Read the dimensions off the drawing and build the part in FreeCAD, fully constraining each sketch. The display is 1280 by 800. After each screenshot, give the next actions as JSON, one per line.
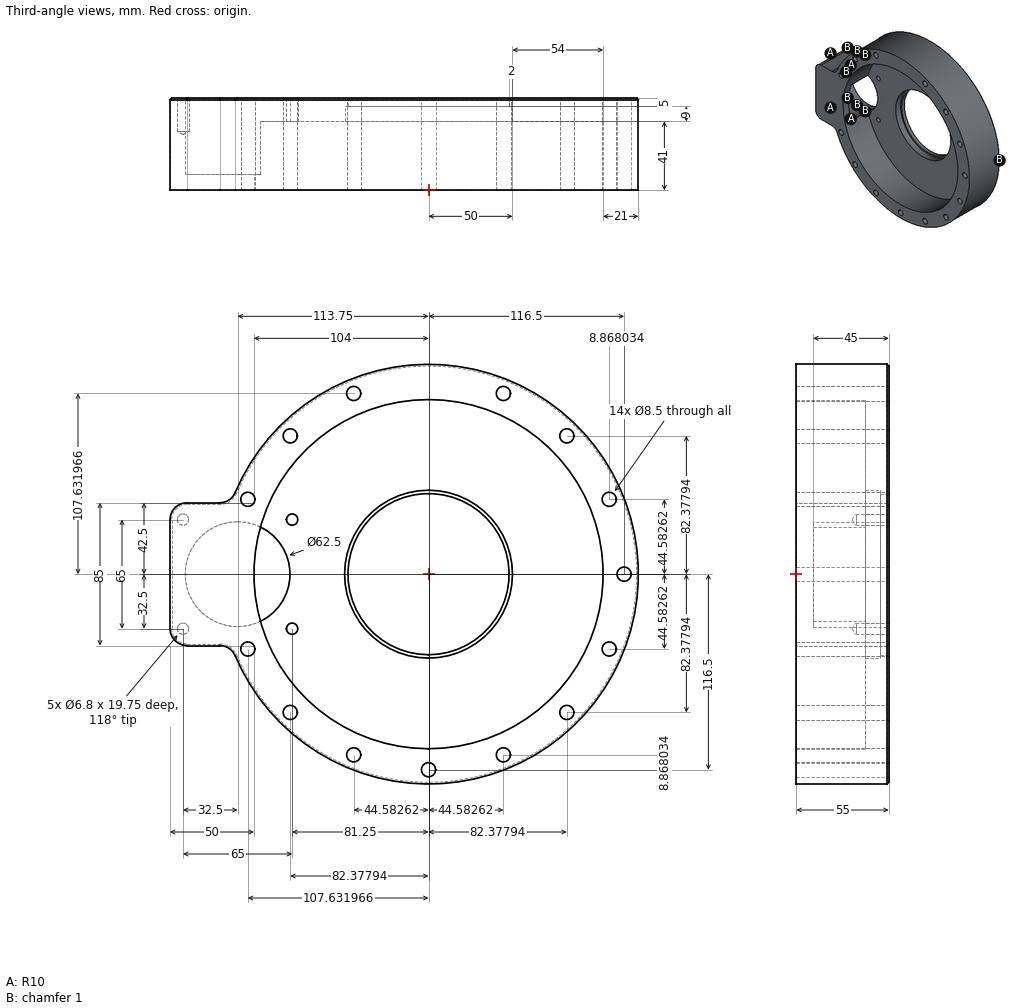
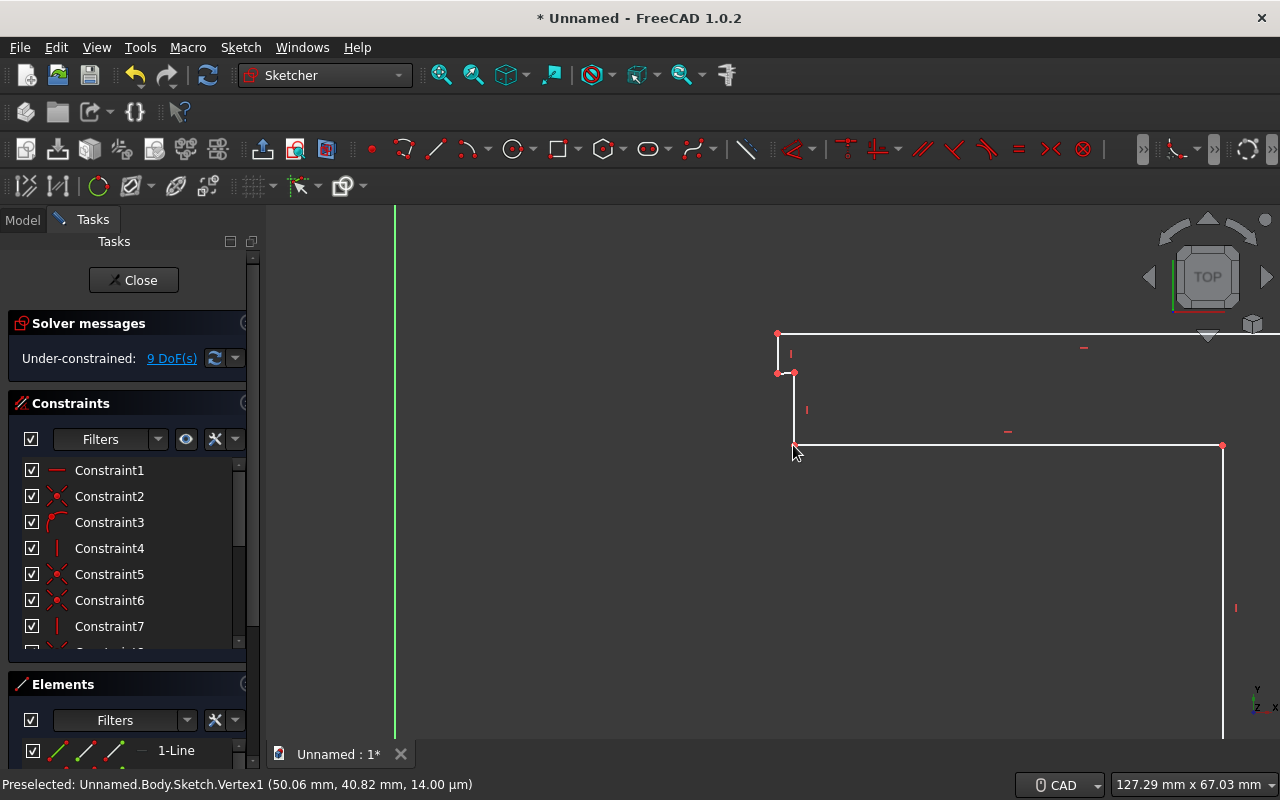
{"action": "scroll", "coordinate": [475, 376], "scroll_direction": "down", "scroll_amount": 3}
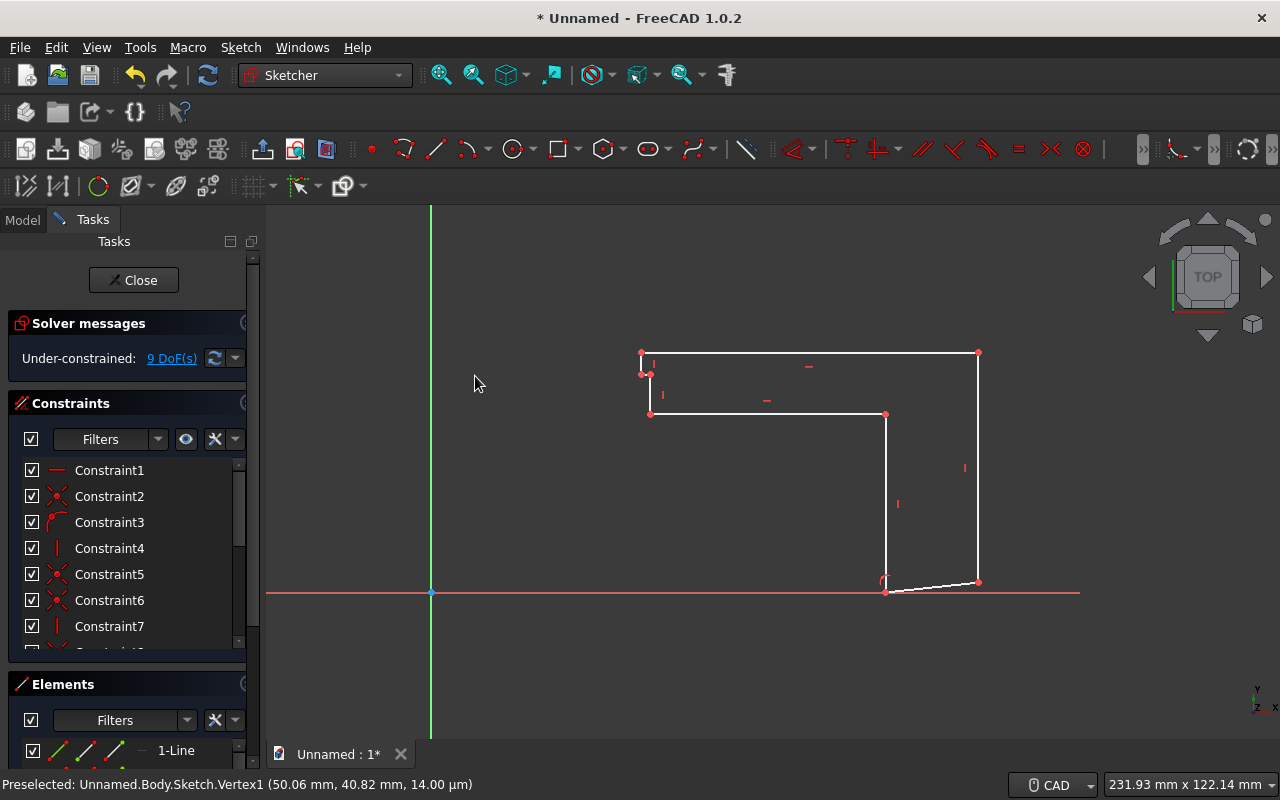
{"action": "scroll", "coordinate": [951, 586], "scroll_direction": "up", "scroll_amount": 4}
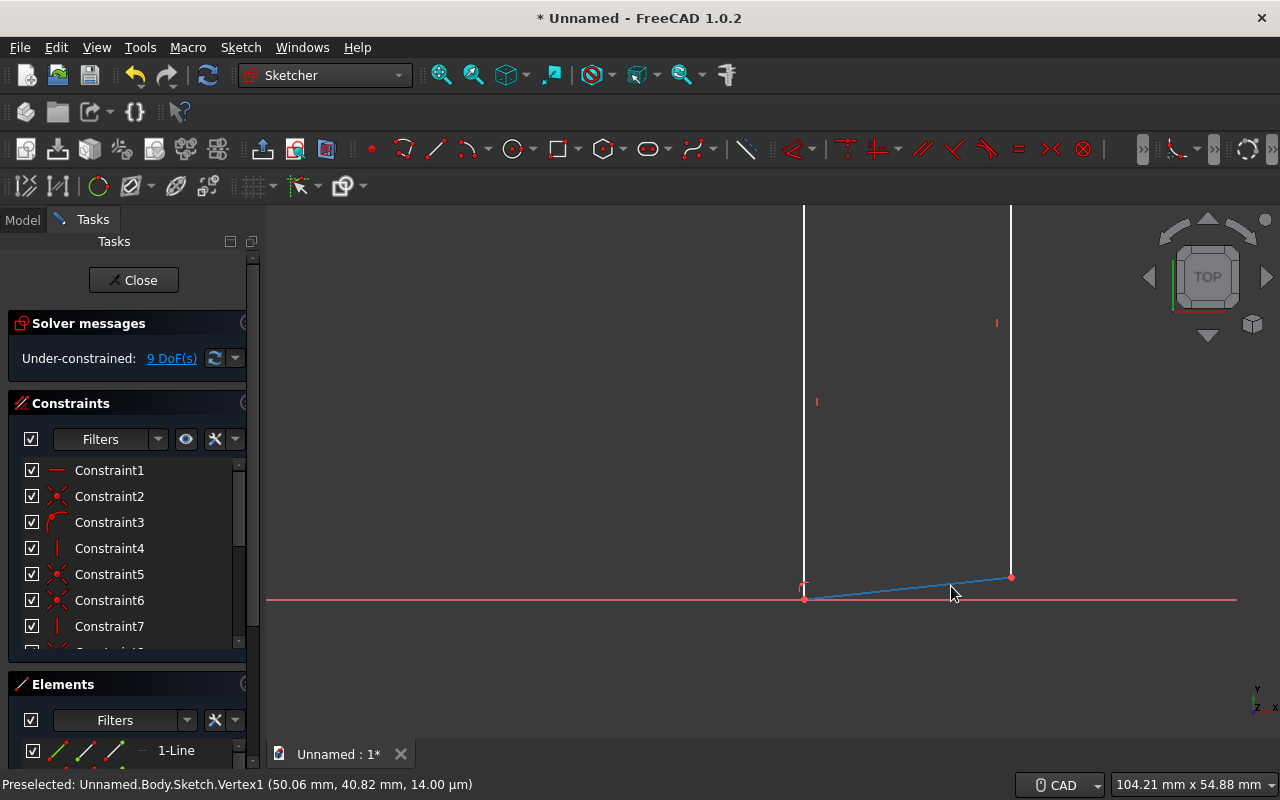
{"action": "left_click", "coordinate": [949, 584]}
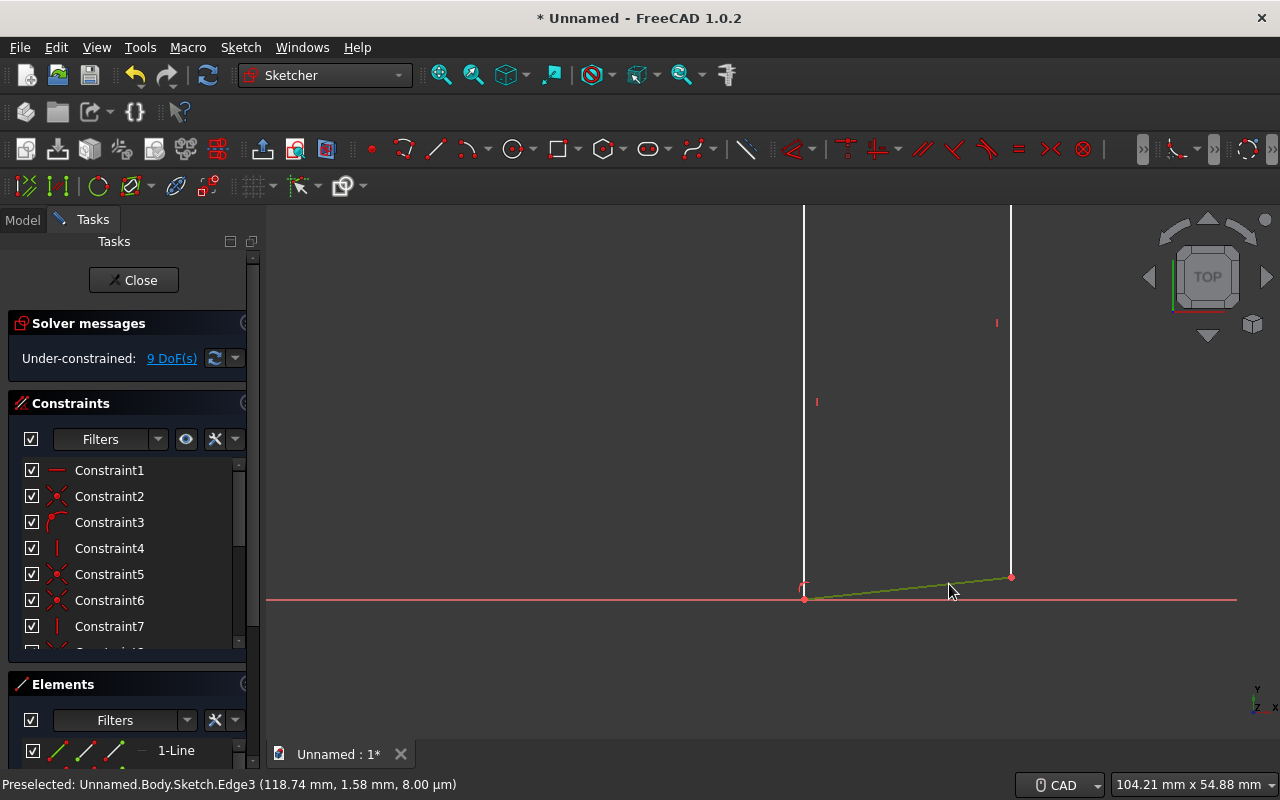
{"action": "key", "text": "h"}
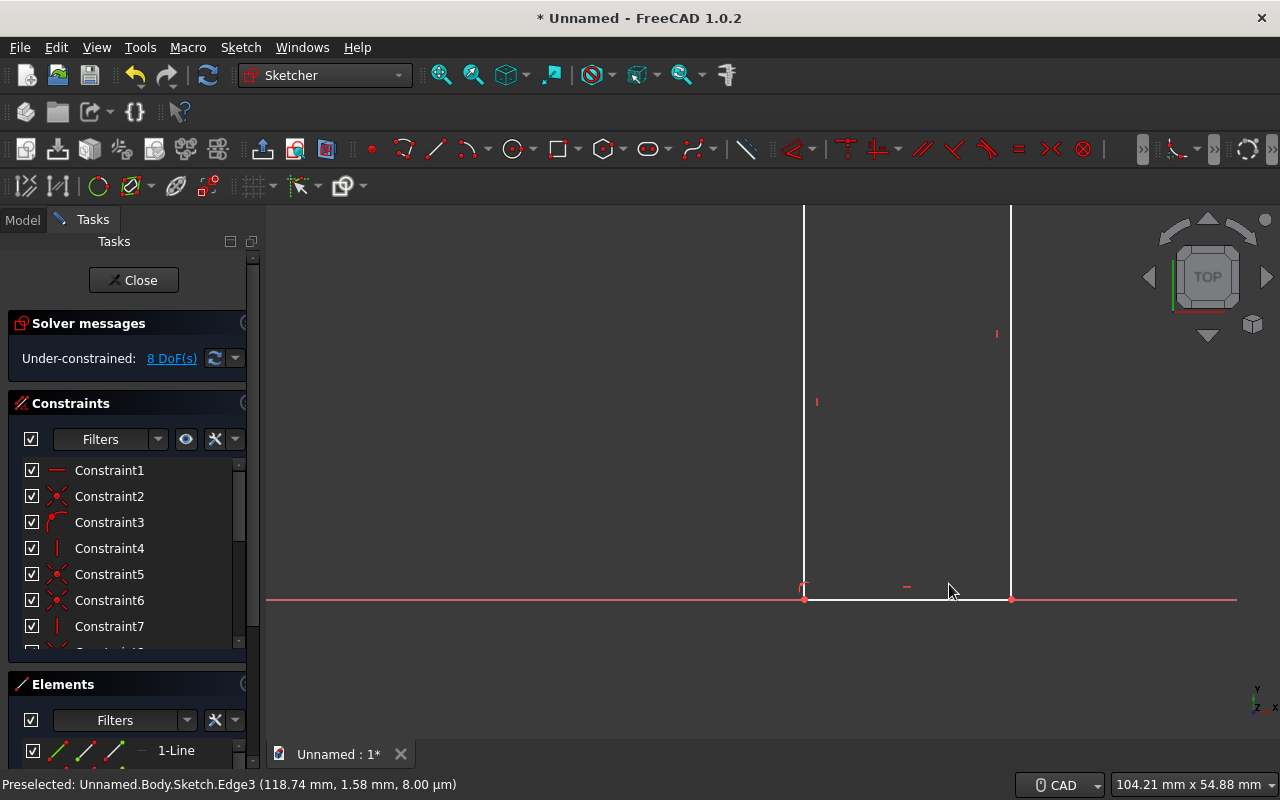
{"action": "scroll", "coordinate": [952, 586], "scroll_direction": "down", "scroll_amount": 4}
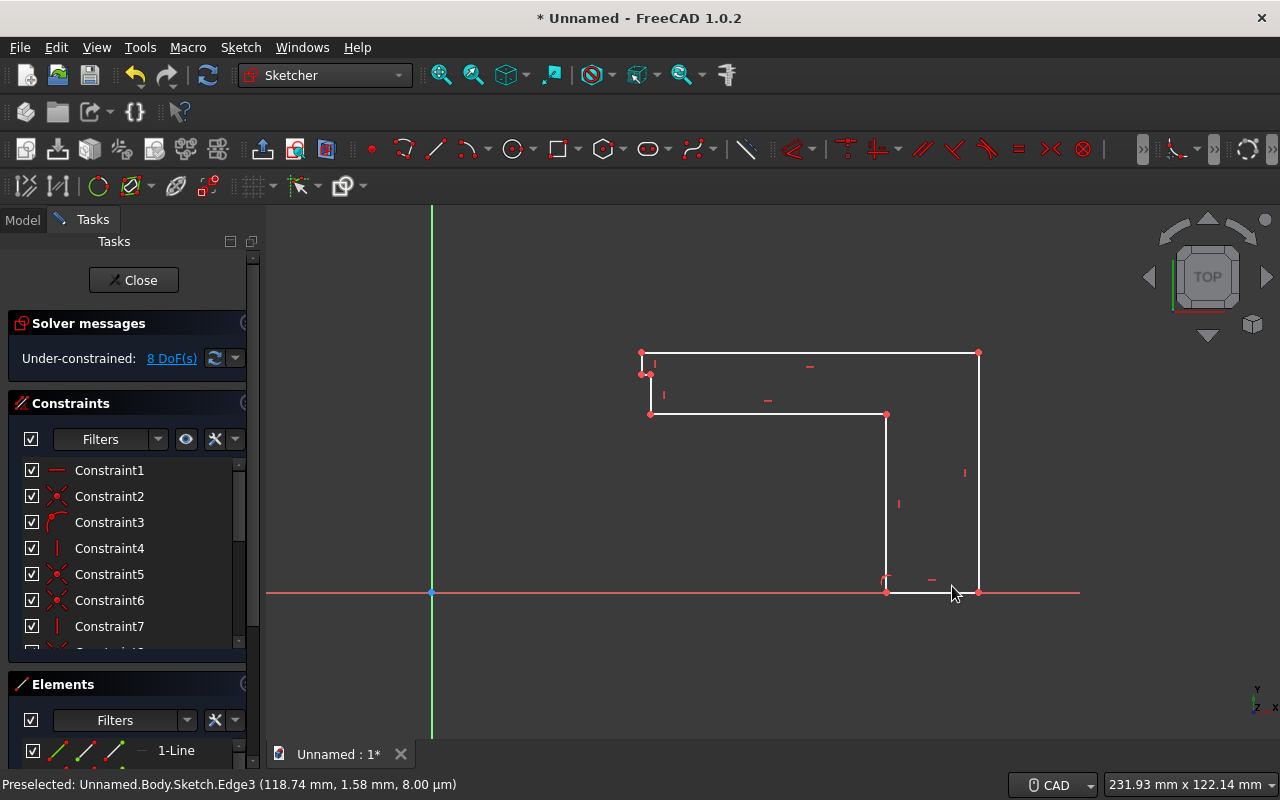
{"action": "scroll", "coordinate": [646, 375], "scroll_direction": "up", "scroll_amount": 6}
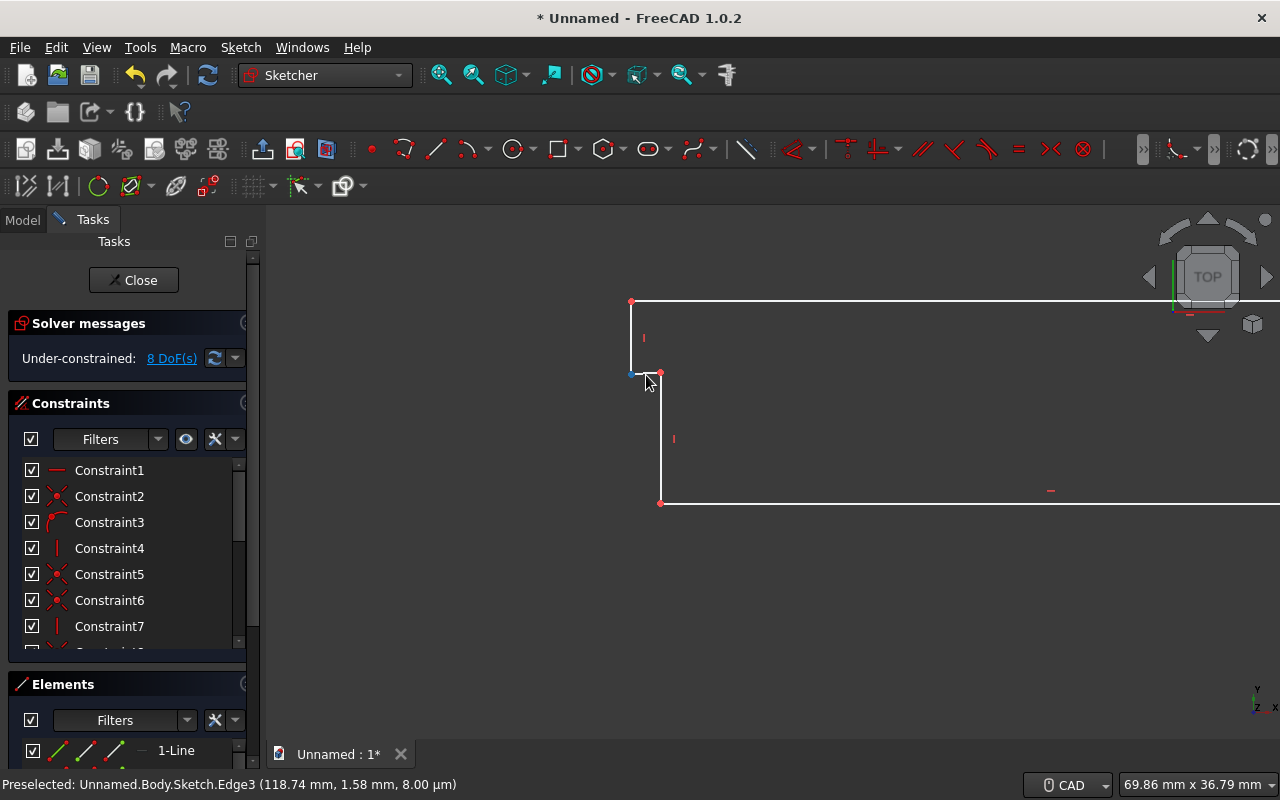
{"action": "left_click", "coordinate": [646, 373]}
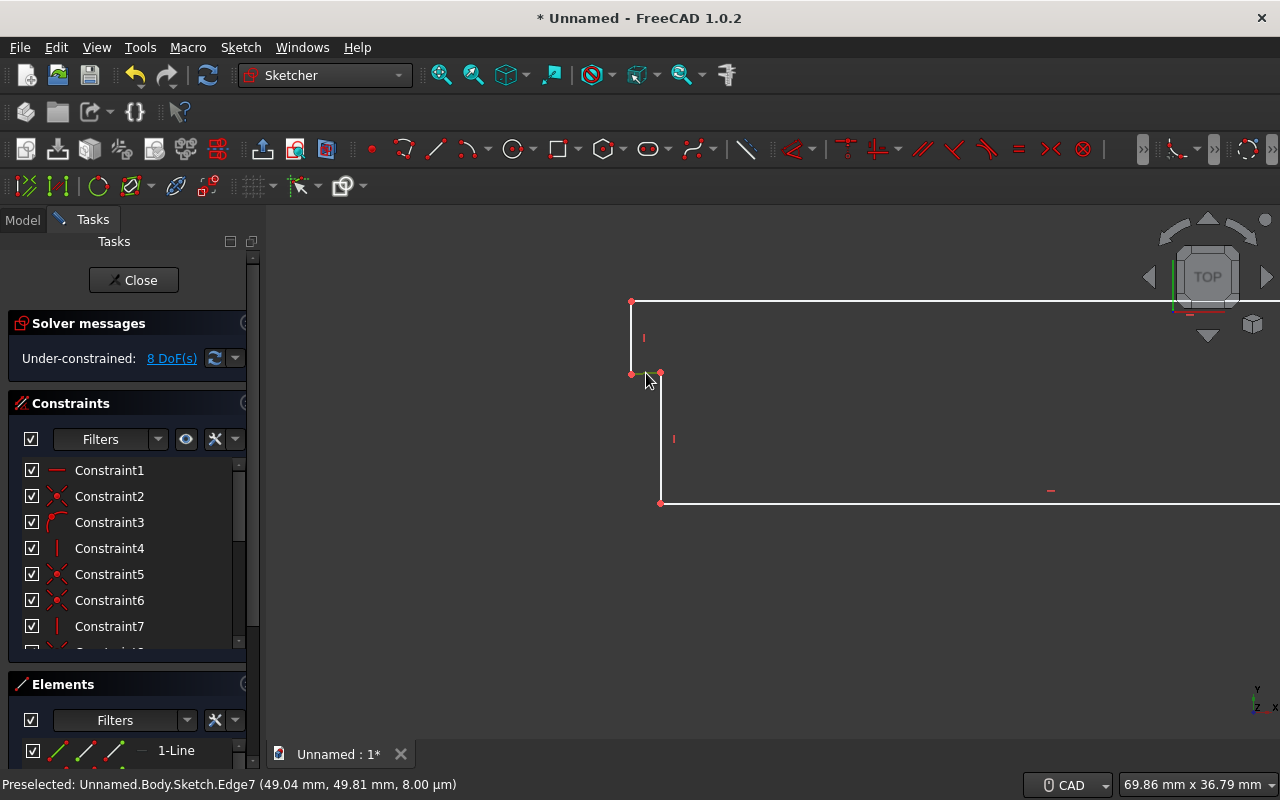
{"action": "left_click", "coordinate": [900, 150]}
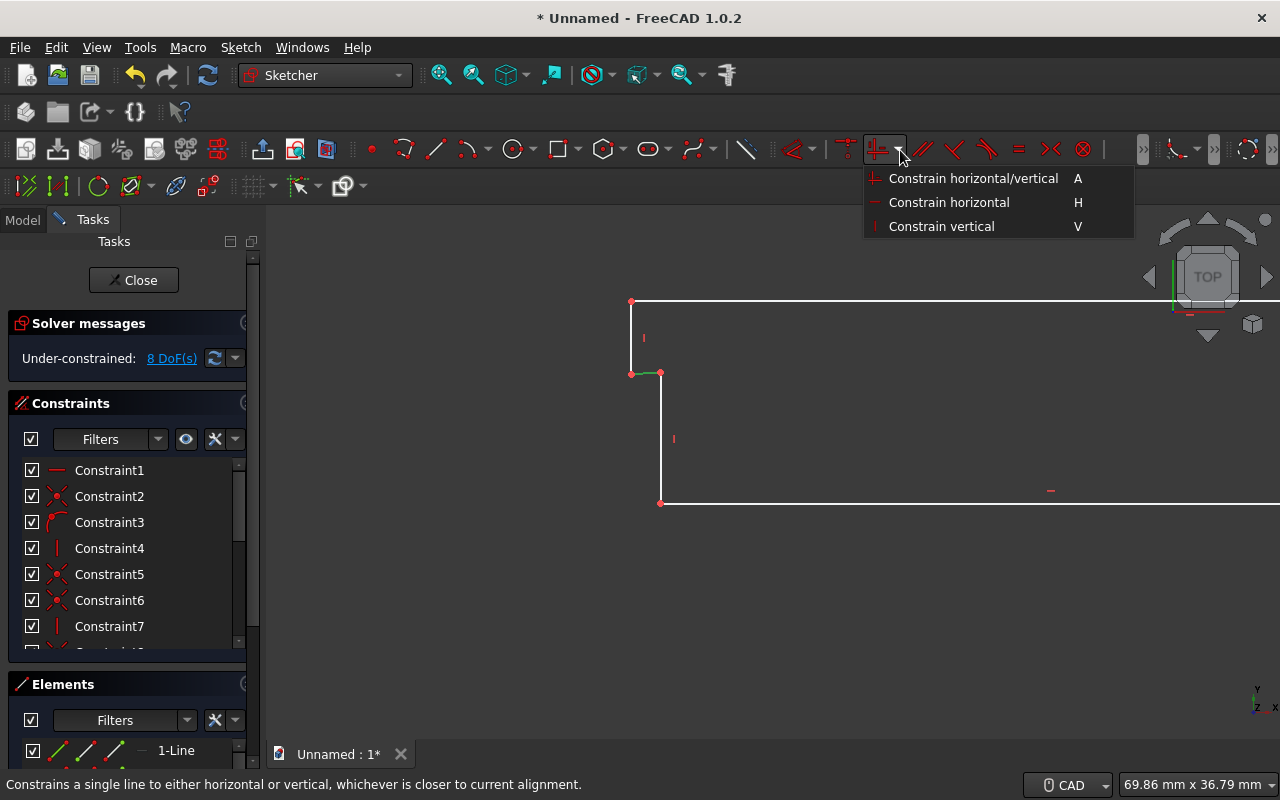
{"action": "left_click", "coordinate": [999, 202]}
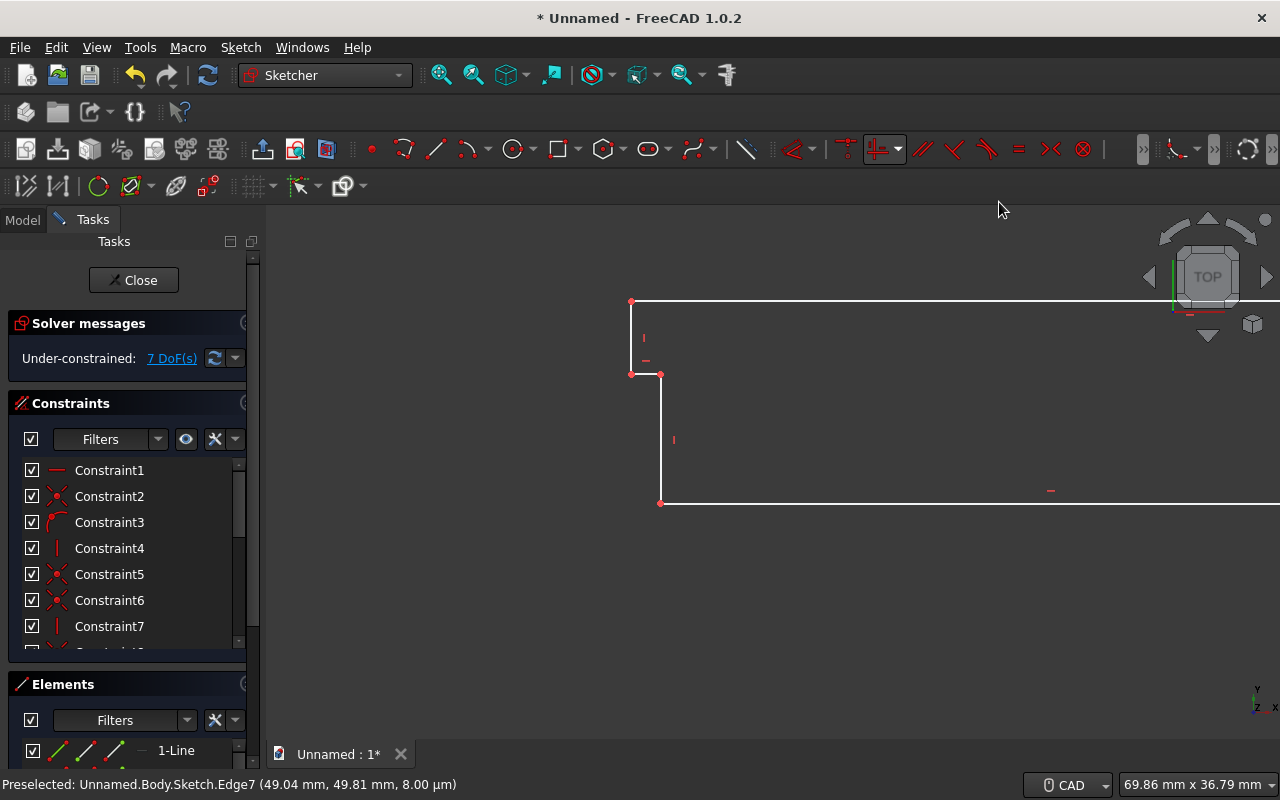
{"action": "left_click", "coordinate": [792, 150]}